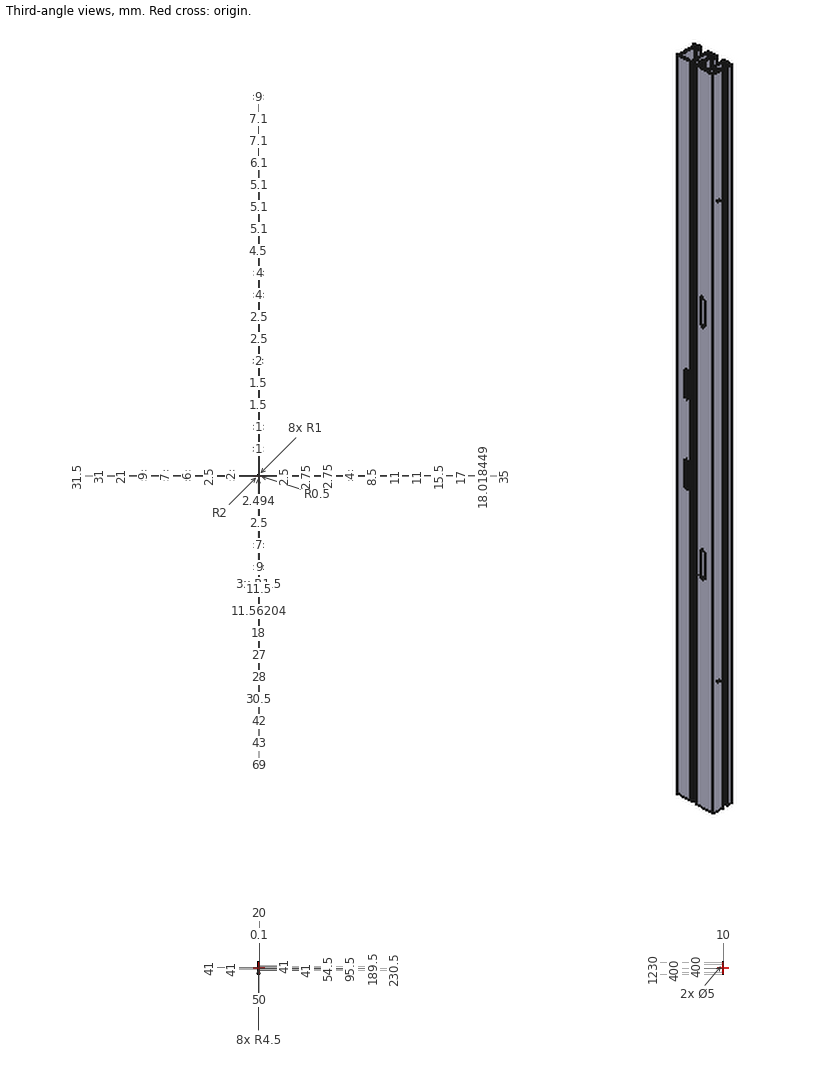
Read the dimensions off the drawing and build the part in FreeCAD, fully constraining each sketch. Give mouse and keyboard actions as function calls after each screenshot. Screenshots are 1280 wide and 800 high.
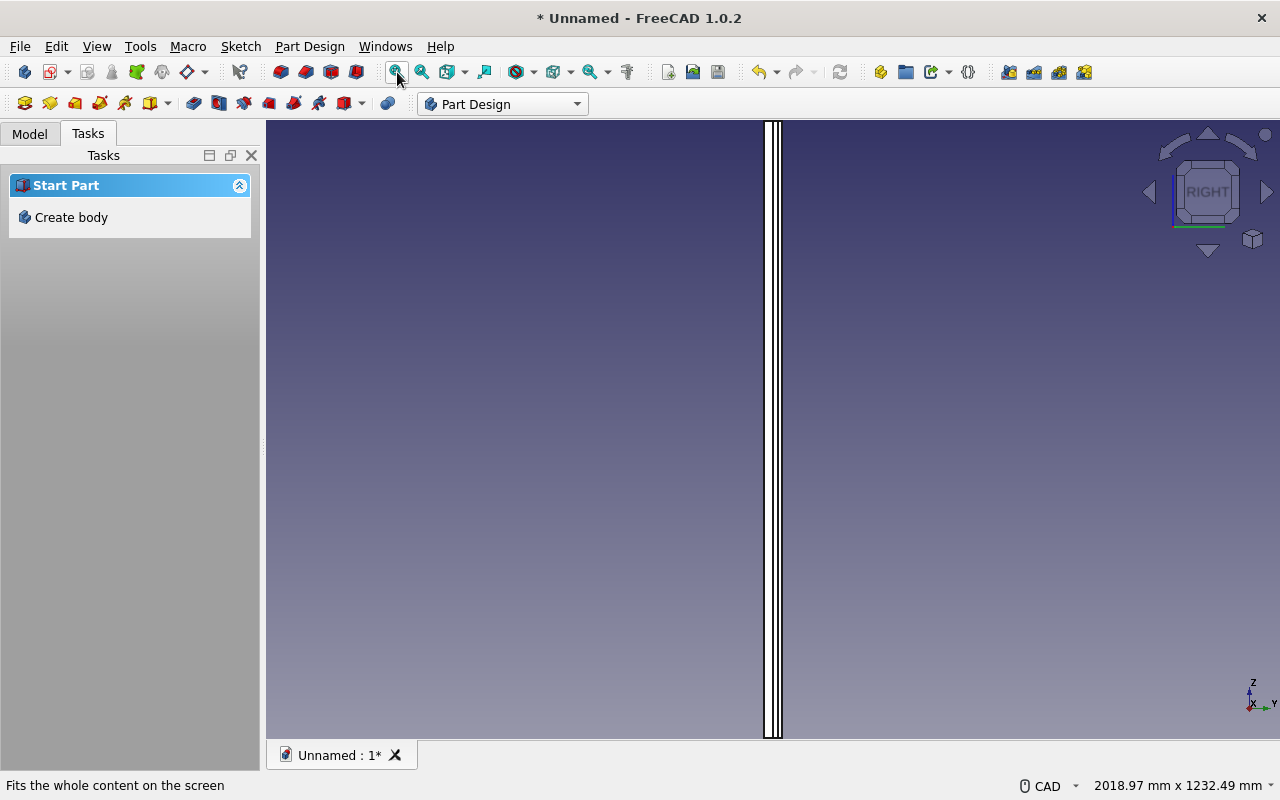
click(30, 134)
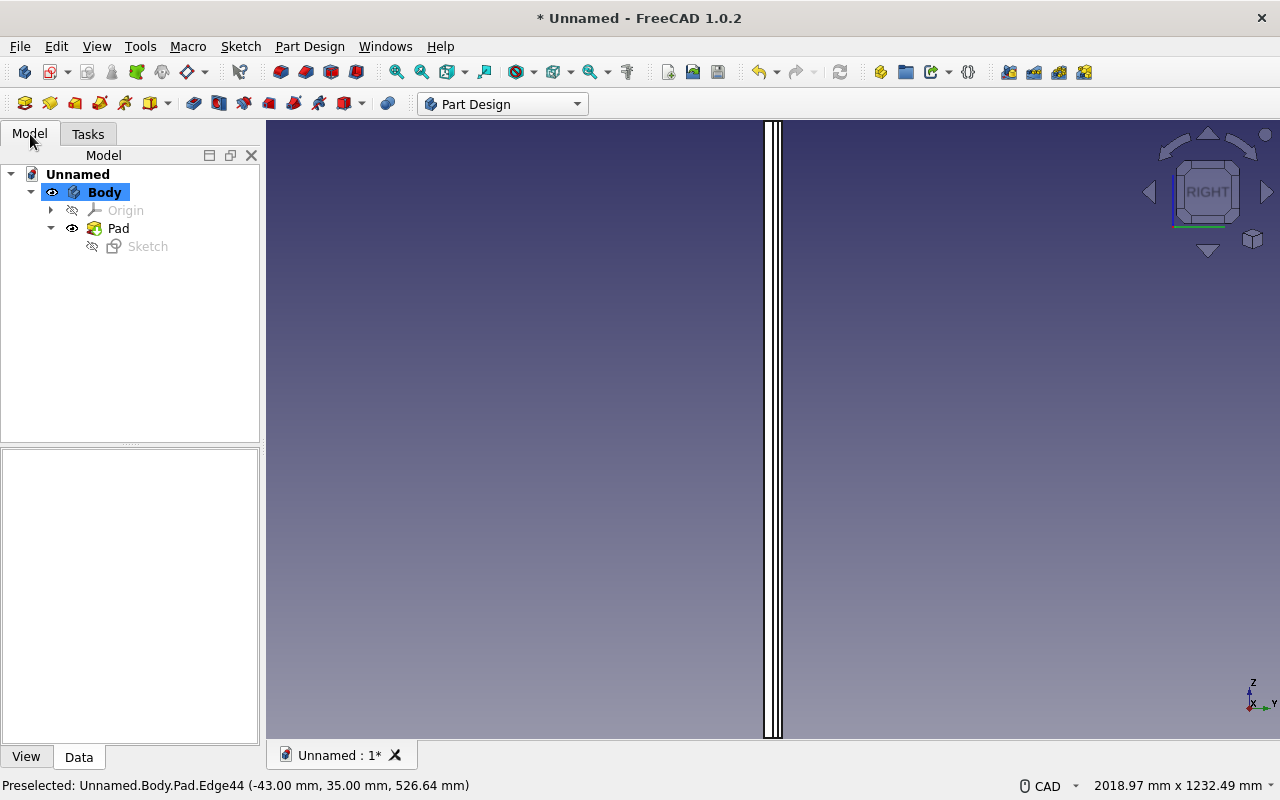
click(51, 210)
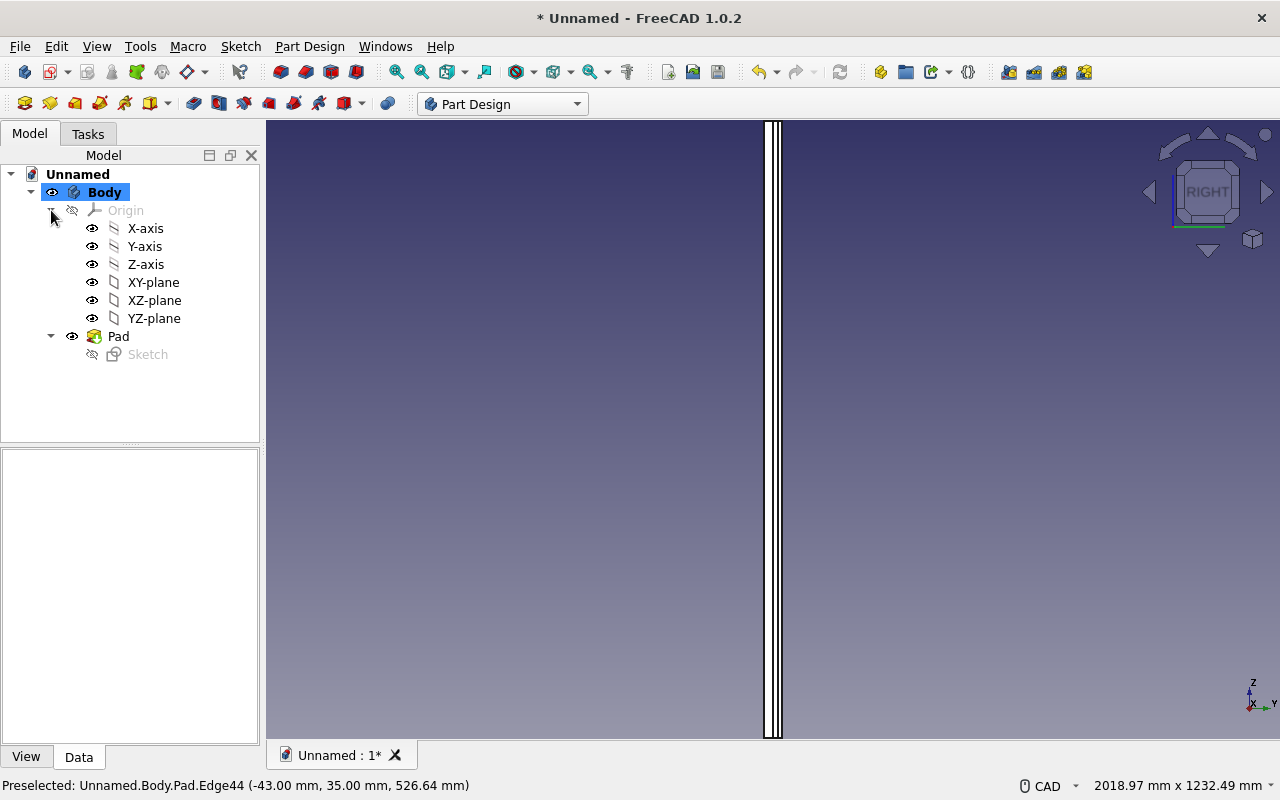
click(137, 300)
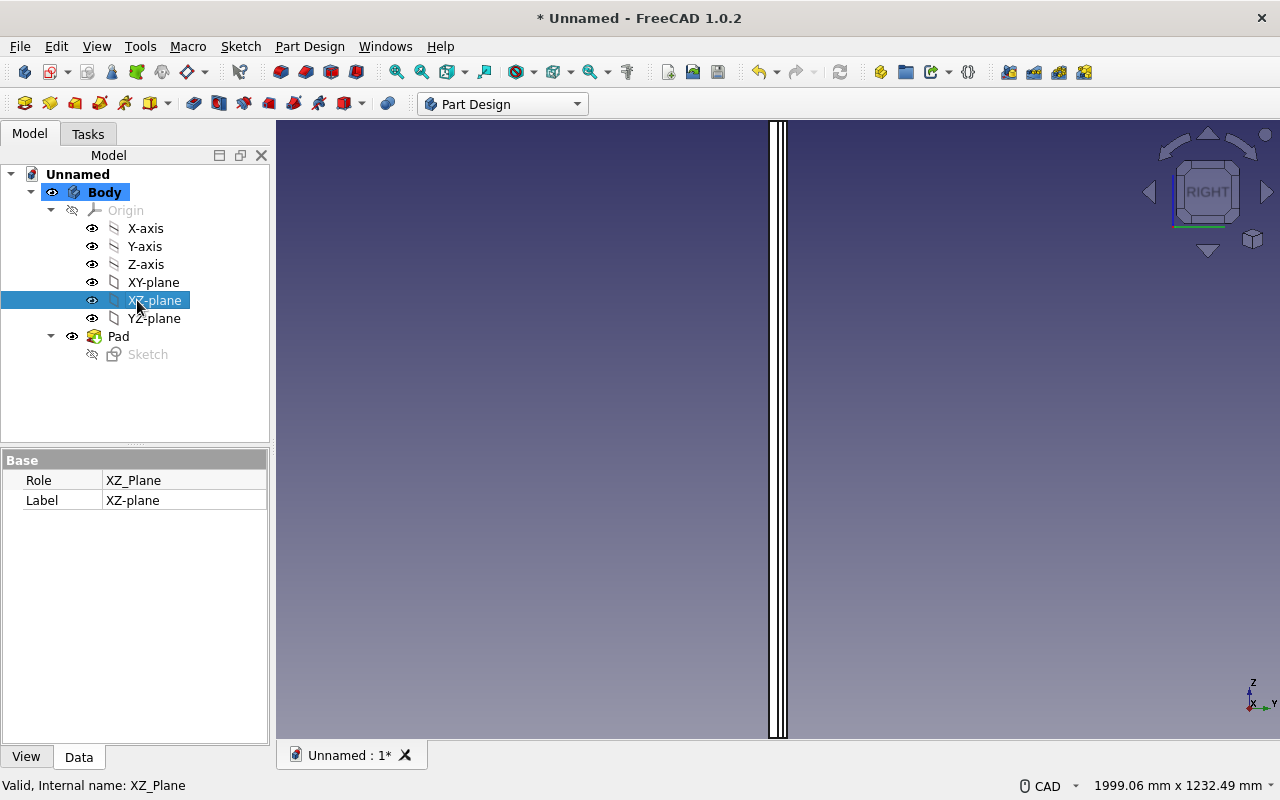
click(186, 72)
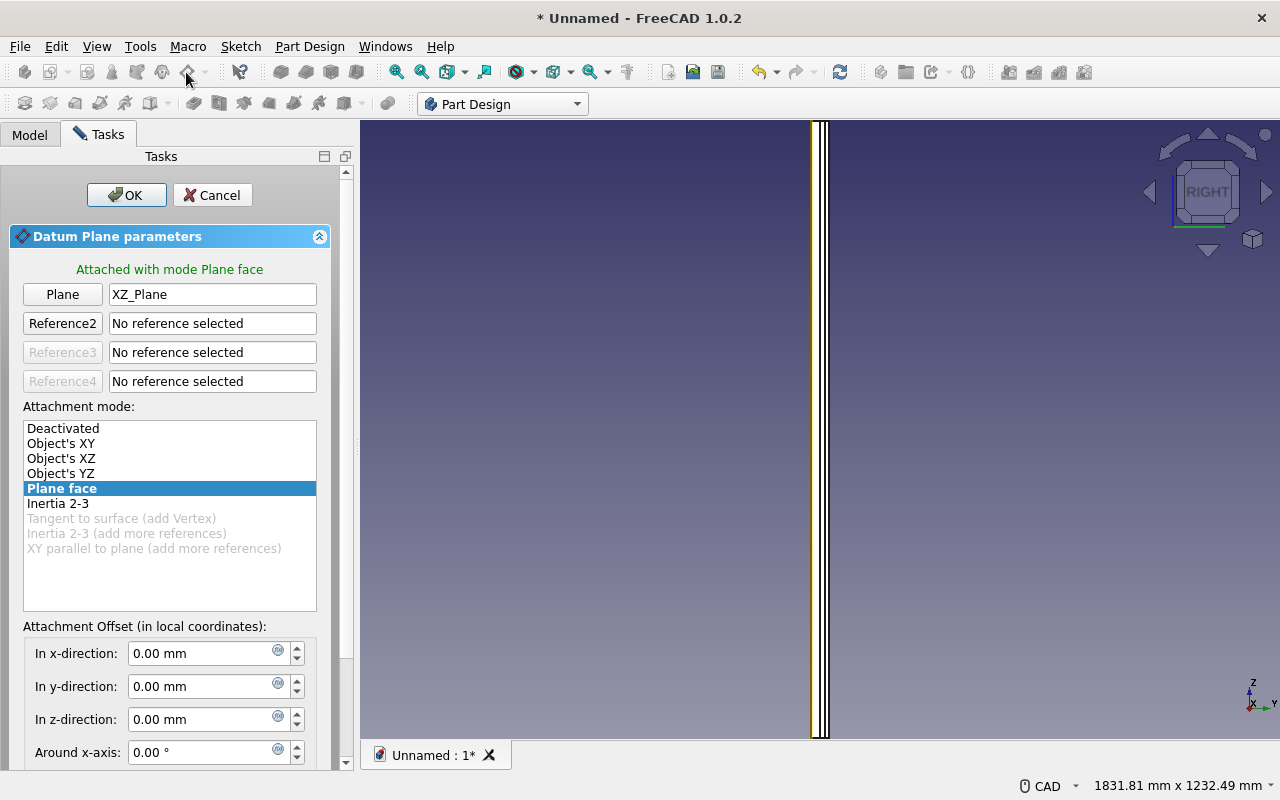
triple_click(210, 720)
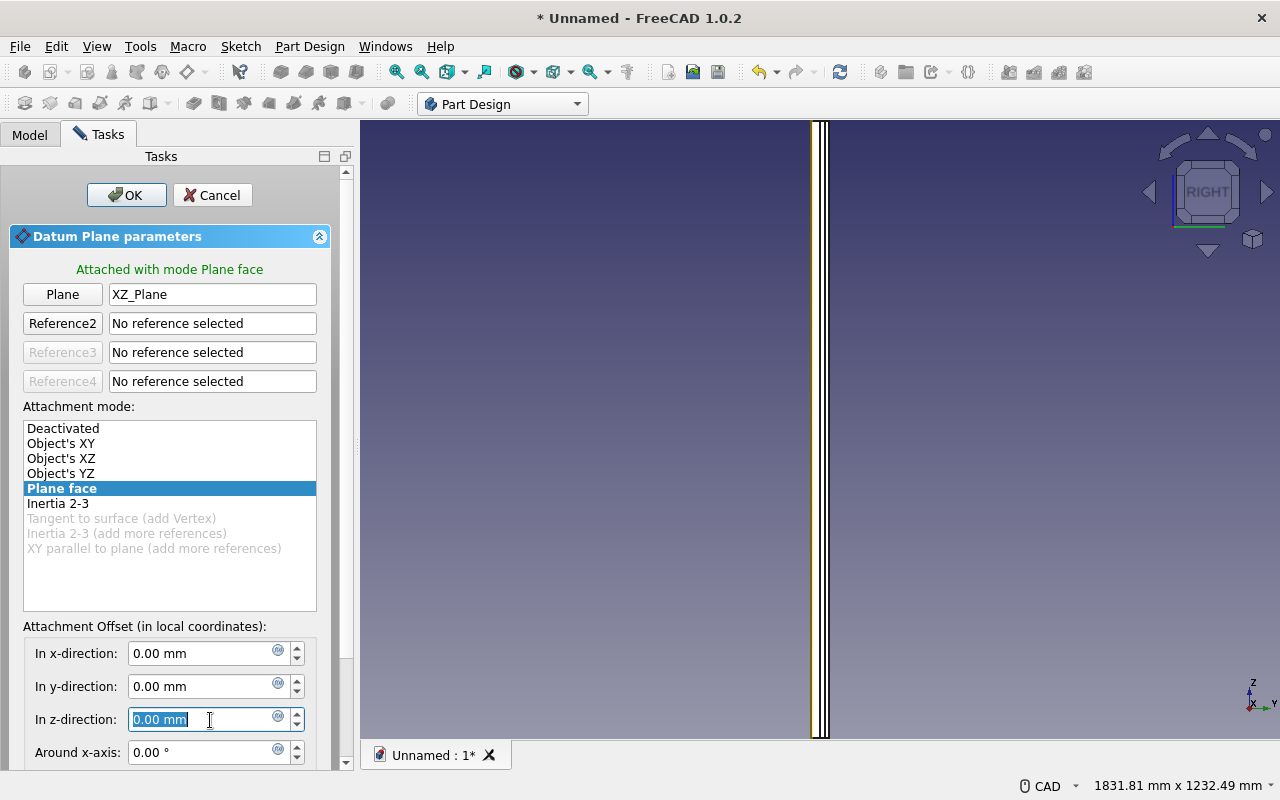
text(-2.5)
key(Tab)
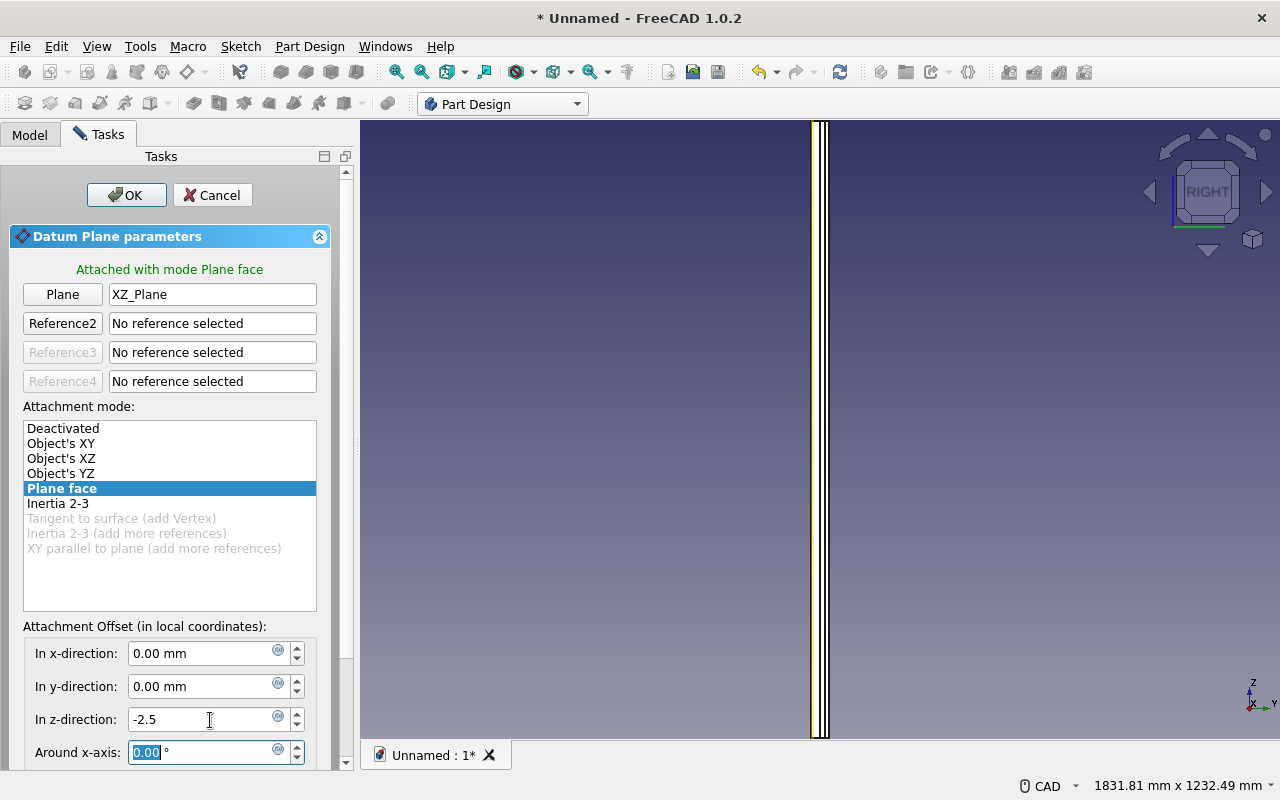
click(127, 195)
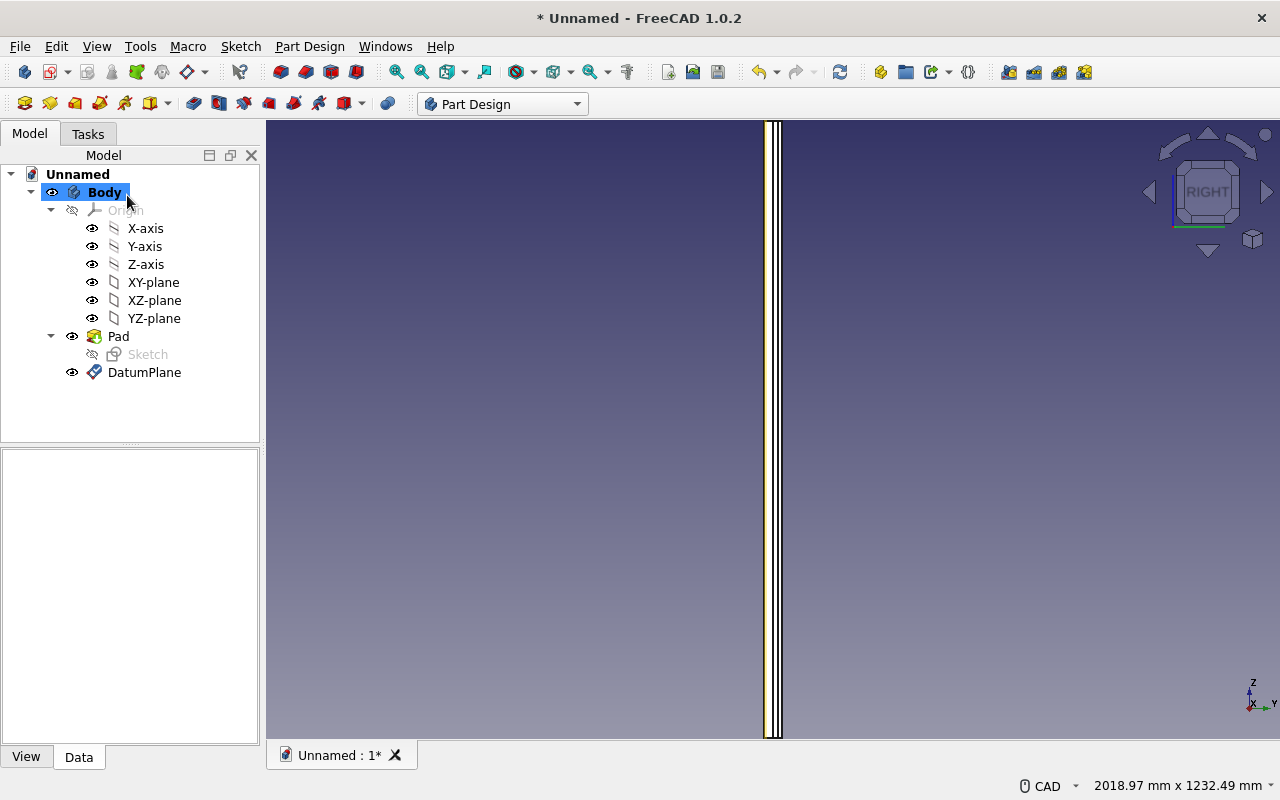
click(117, 372)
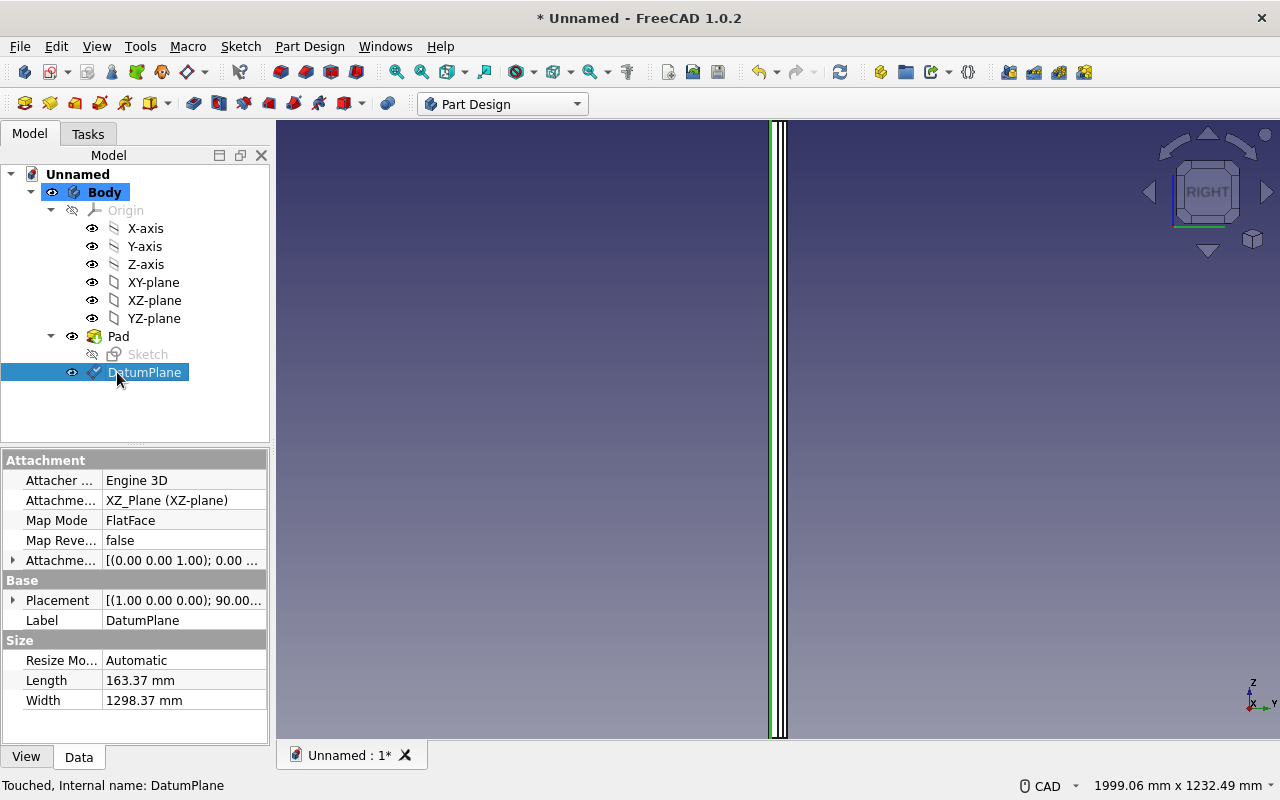
click(50, 72)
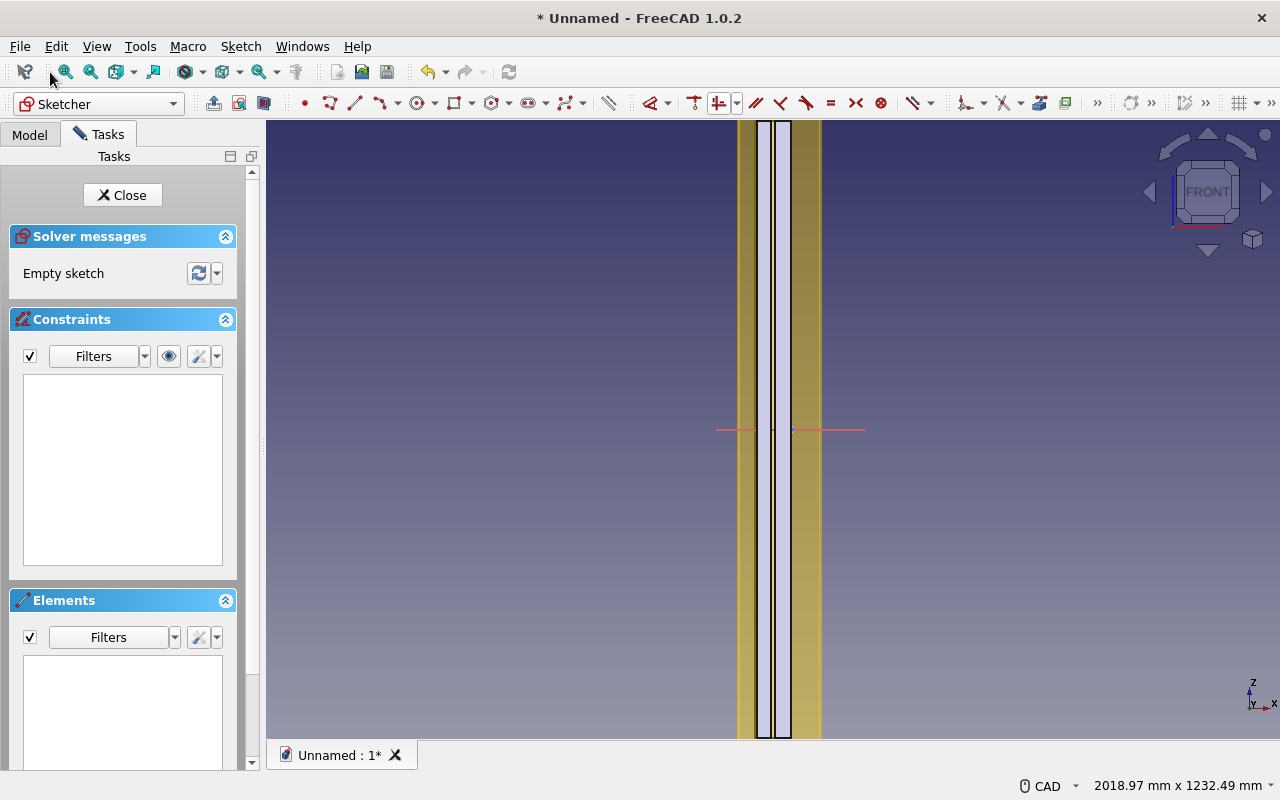
click(264, 104)